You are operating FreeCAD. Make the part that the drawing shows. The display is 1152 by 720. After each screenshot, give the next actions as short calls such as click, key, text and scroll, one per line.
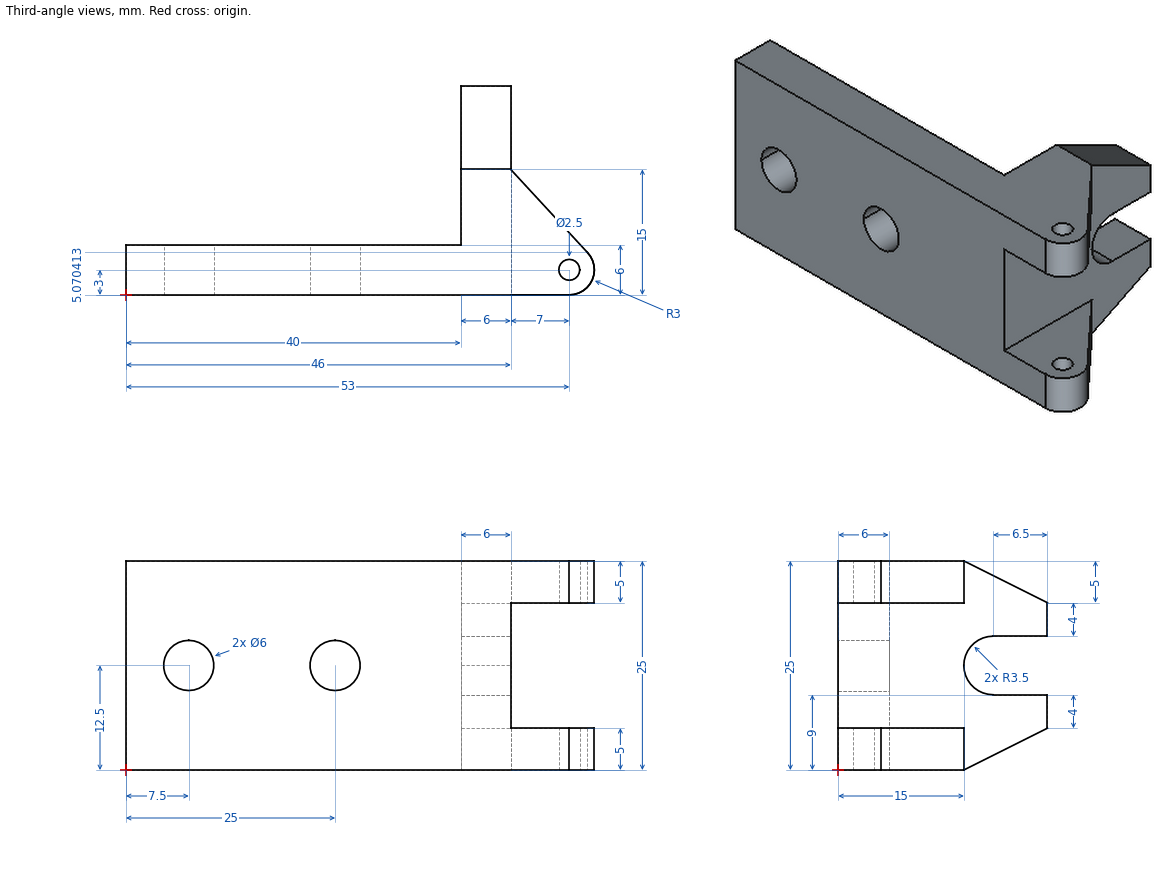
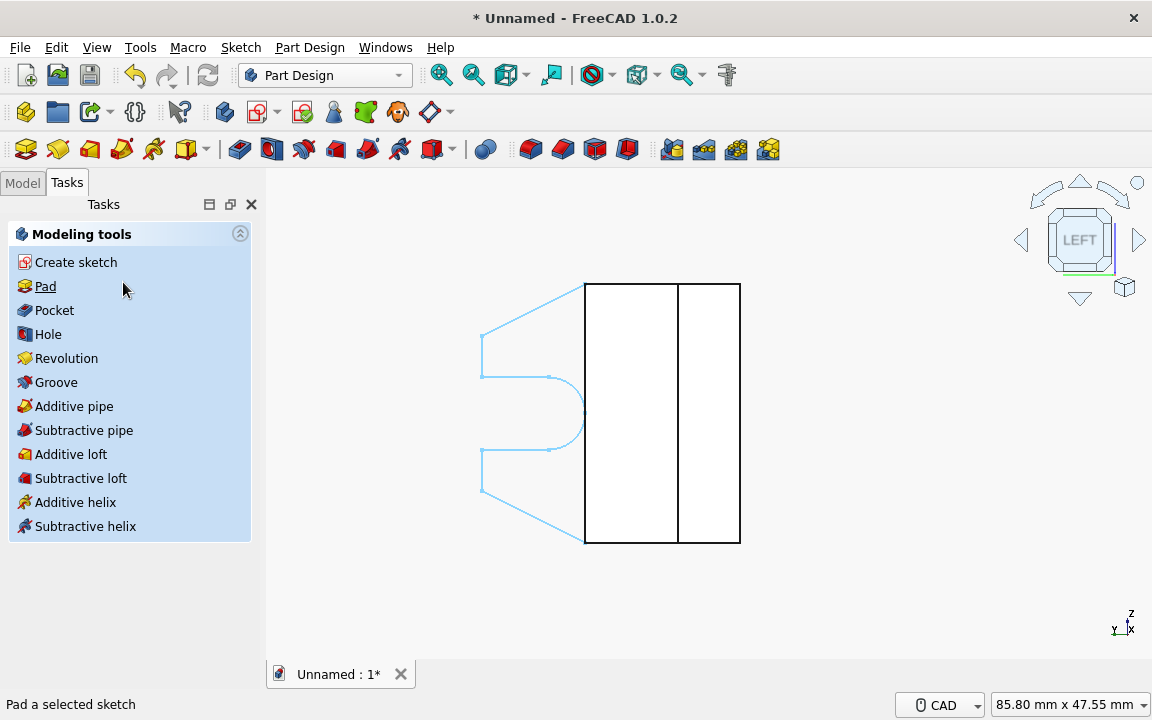
click(26, 150)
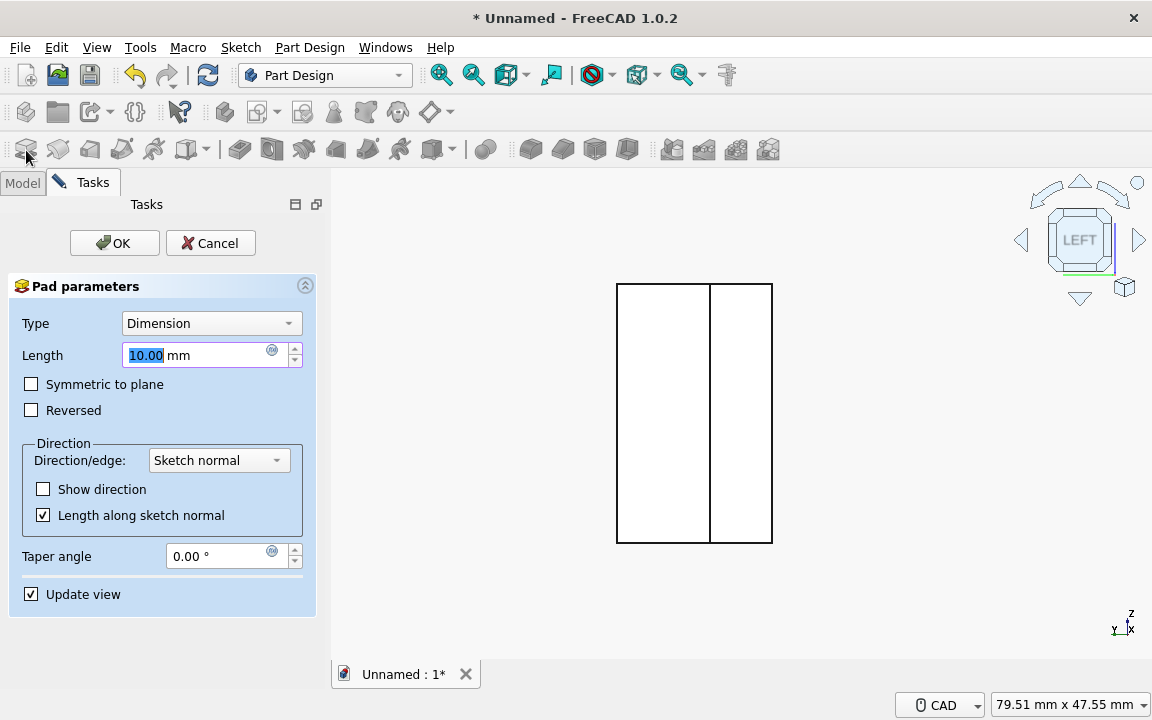
text(6)
key(Tab)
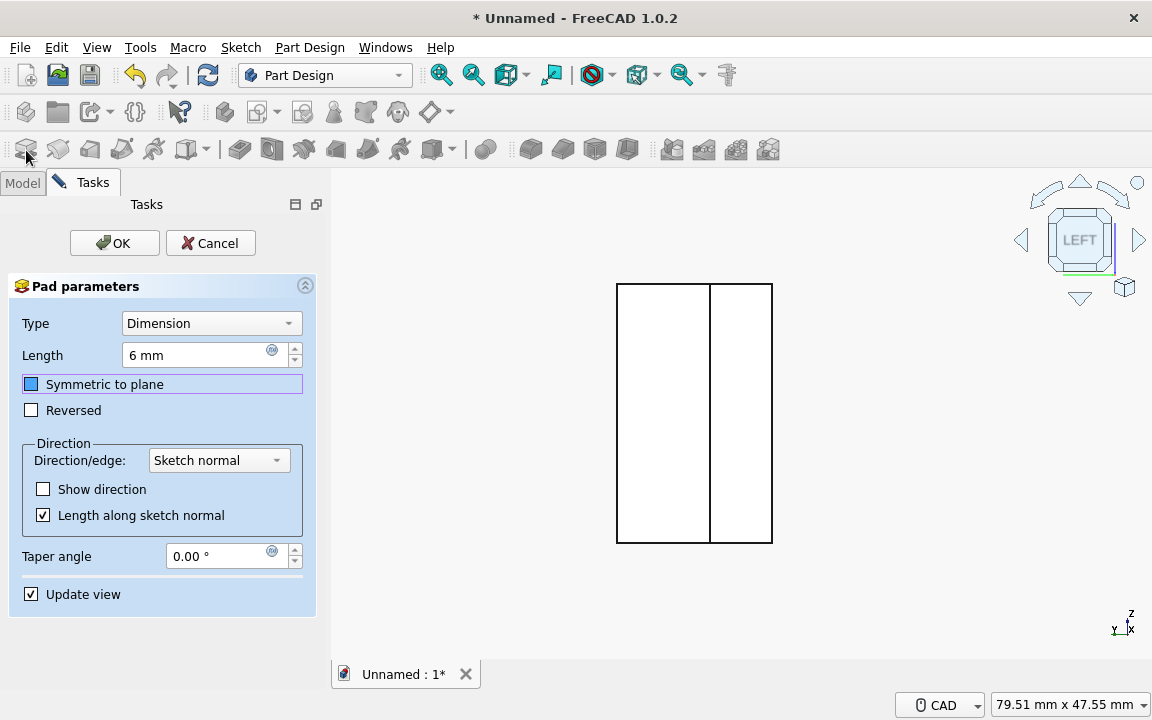
click(30, 410)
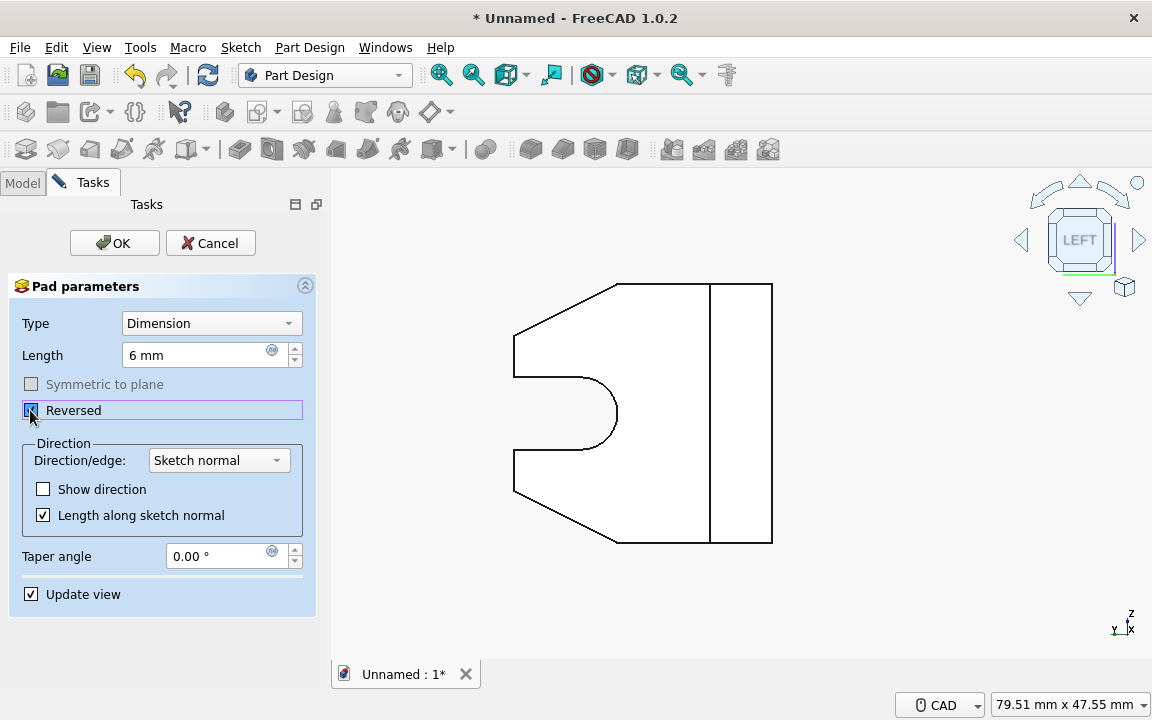
click(115, 243)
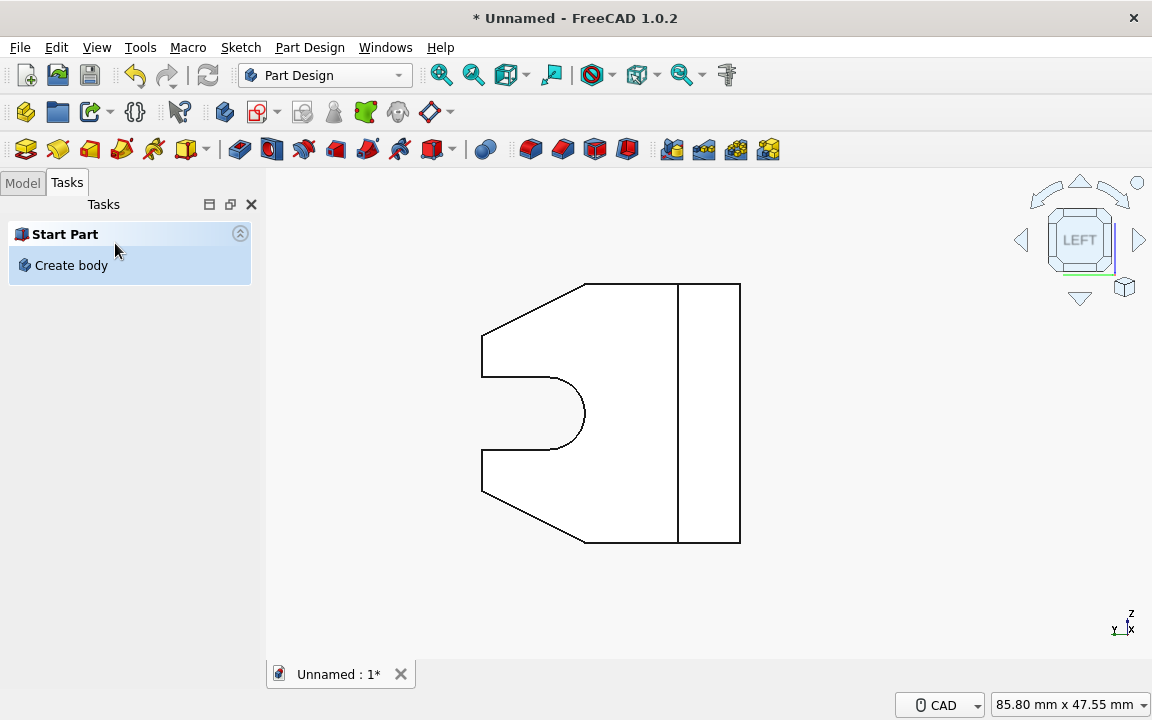
key(0)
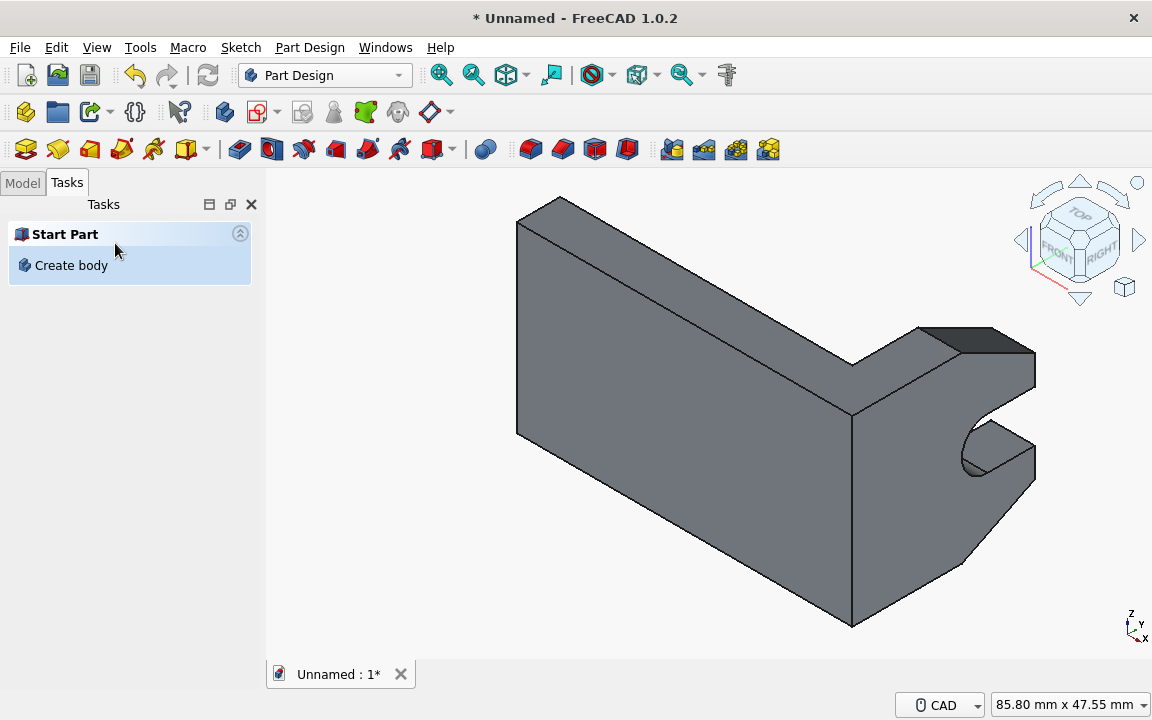
key(v)
key(f)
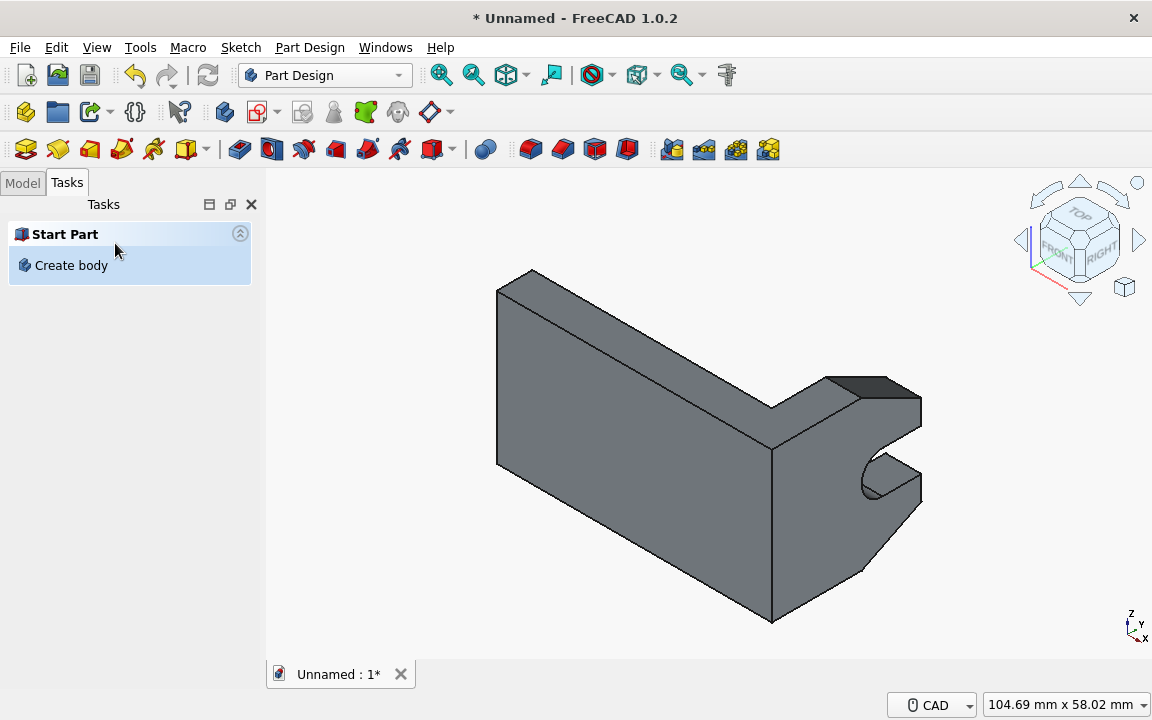
click(771, 426)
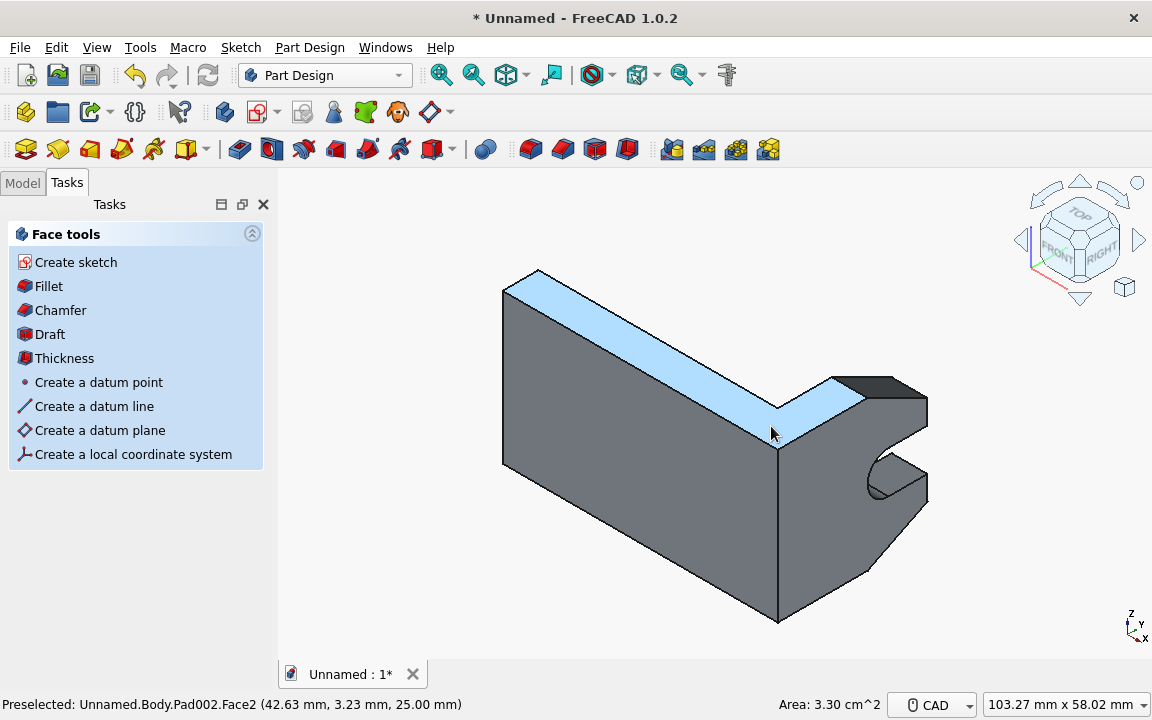
click(258, 112)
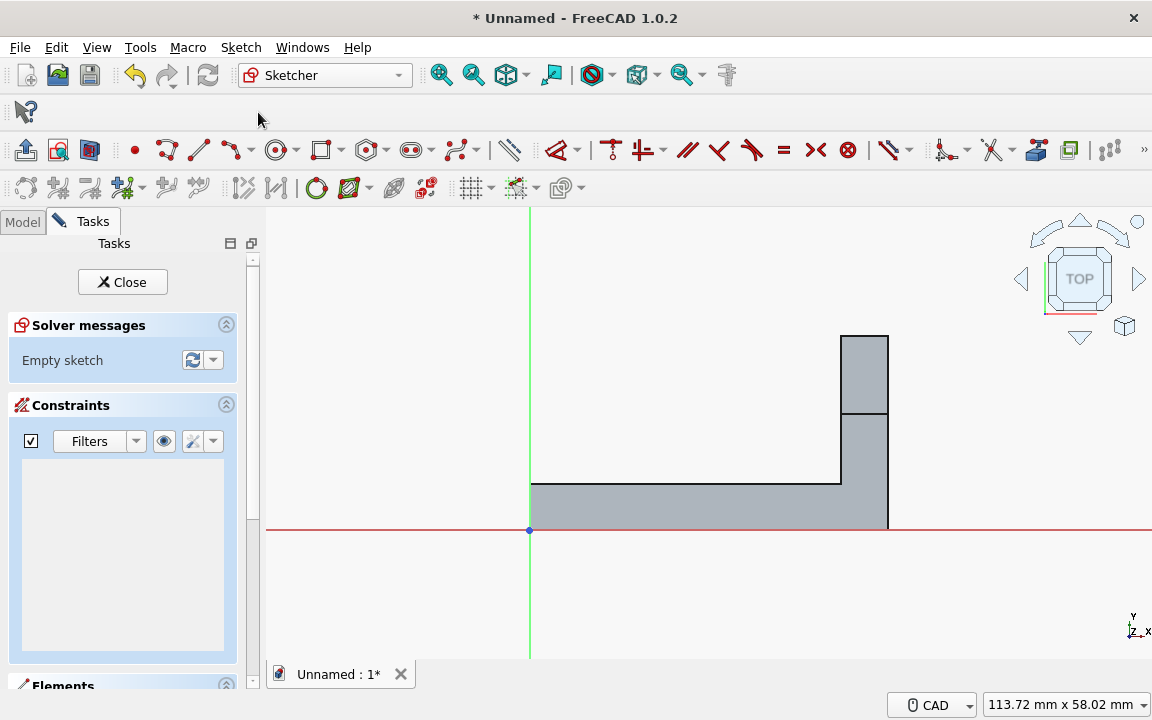
scroll(987, 504, up, 4)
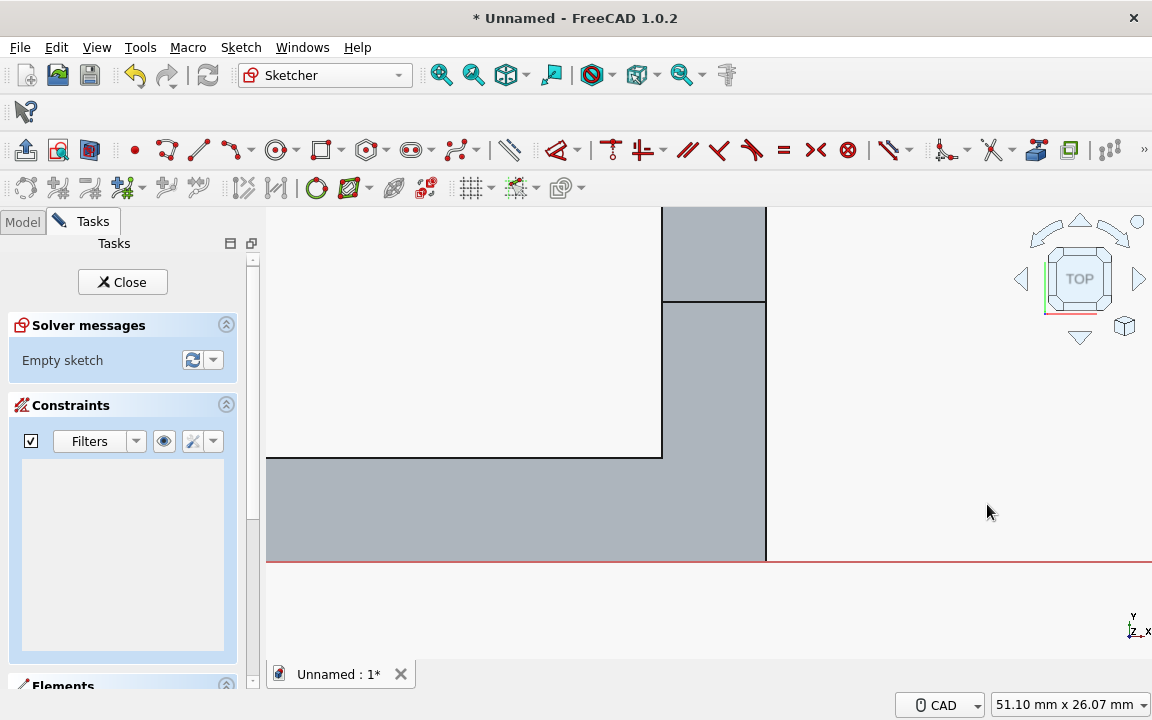
key(g)
key(m)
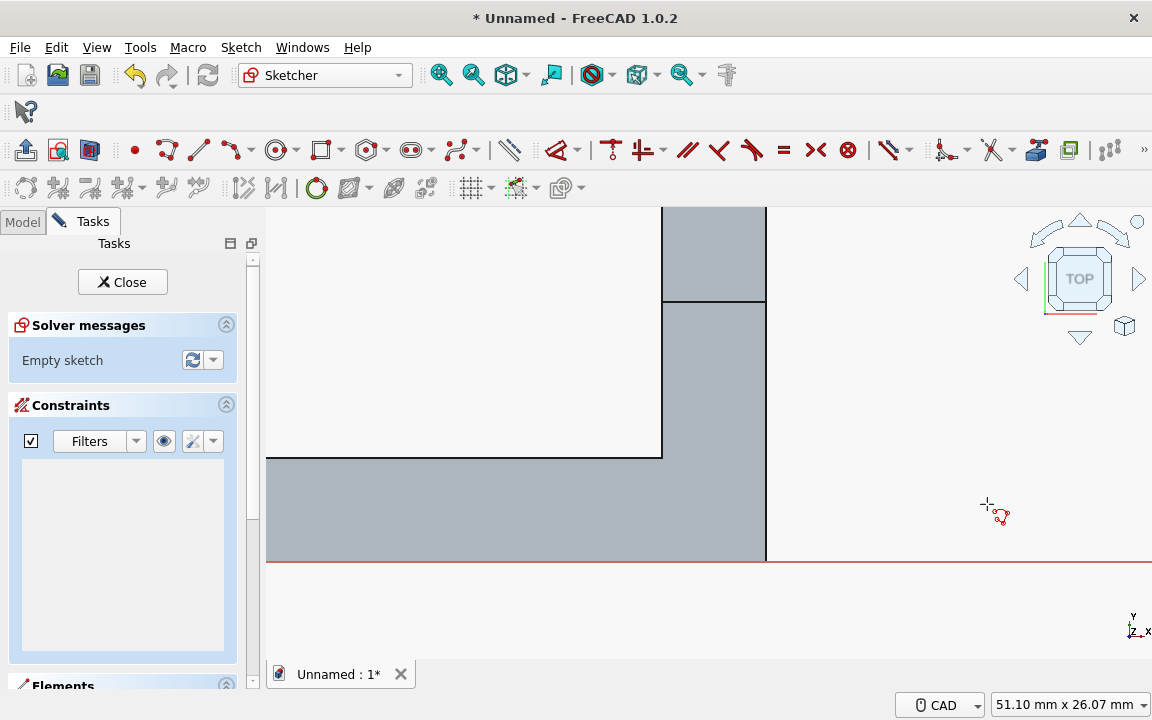
click(925, 474)
click(766, 302)
click(766, 562)
click(887, 553)
right_click(887, 553)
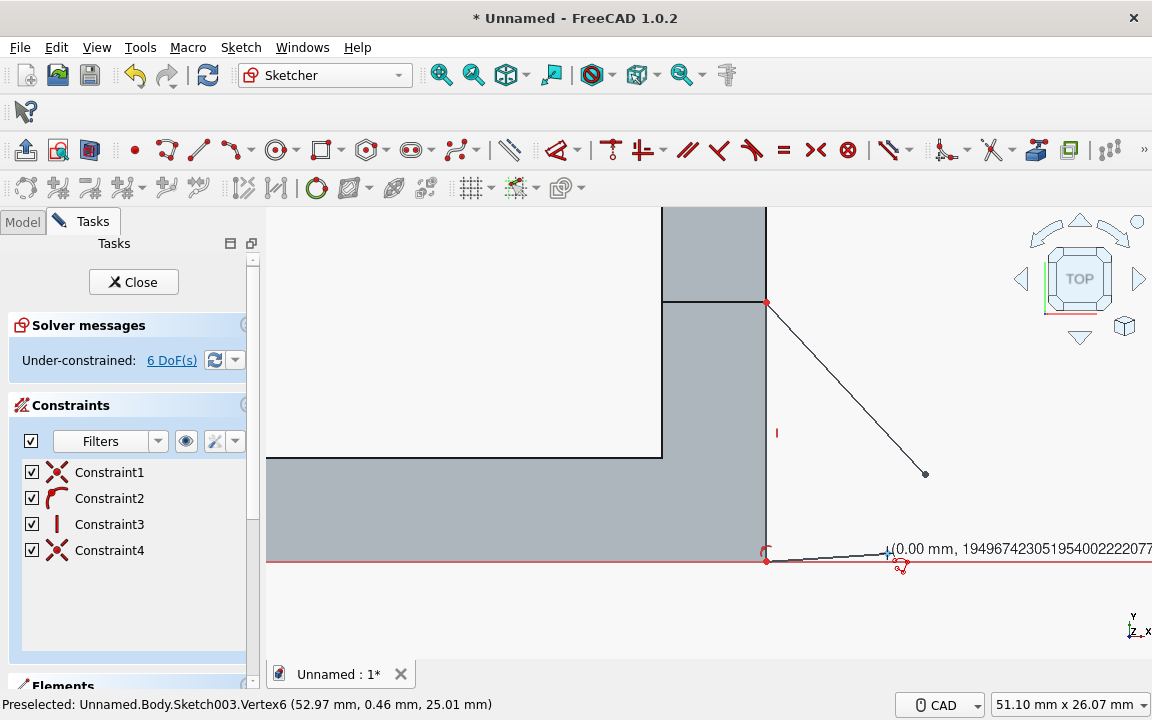
click(232, 150)